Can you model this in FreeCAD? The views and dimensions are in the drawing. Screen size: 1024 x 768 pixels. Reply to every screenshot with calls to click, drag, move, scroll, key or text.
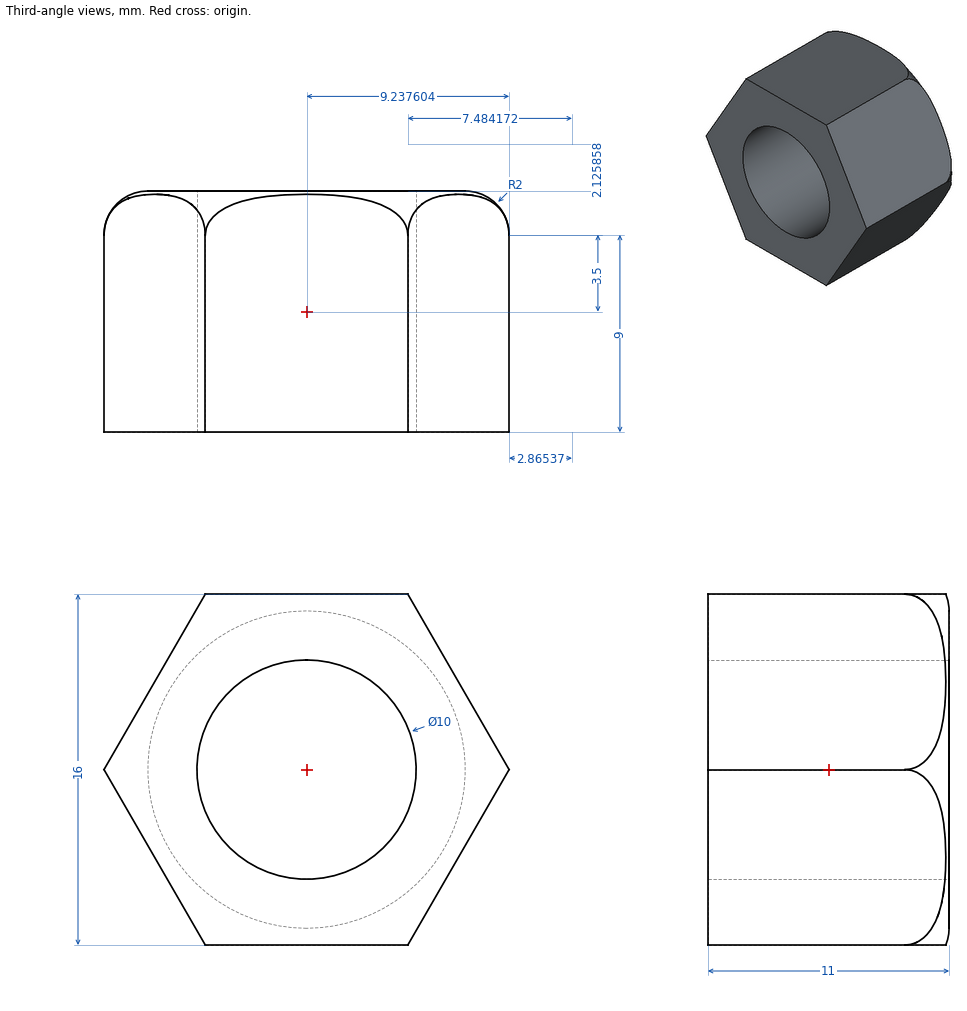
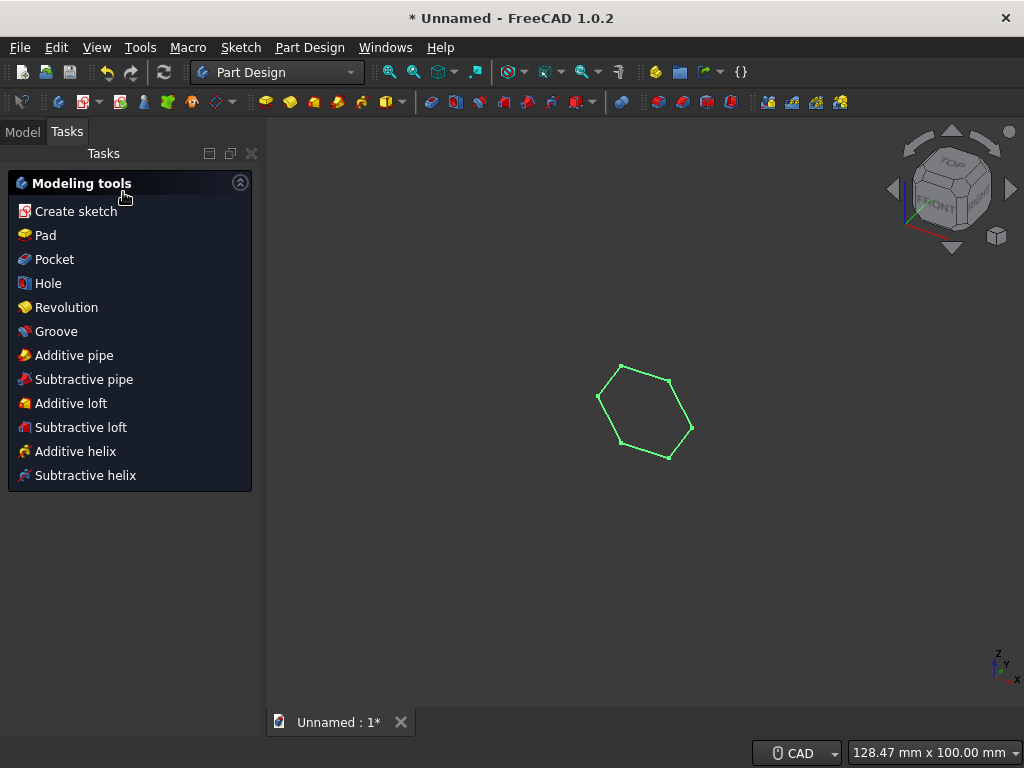
click(266, 102)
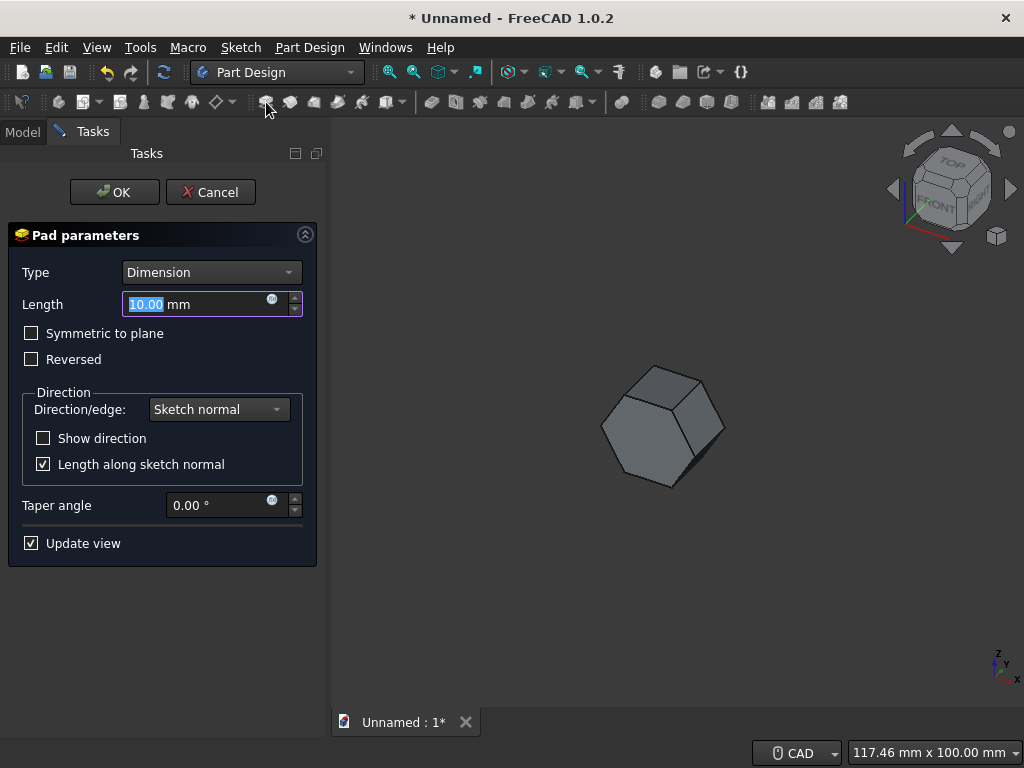
text(11)
key(Tab)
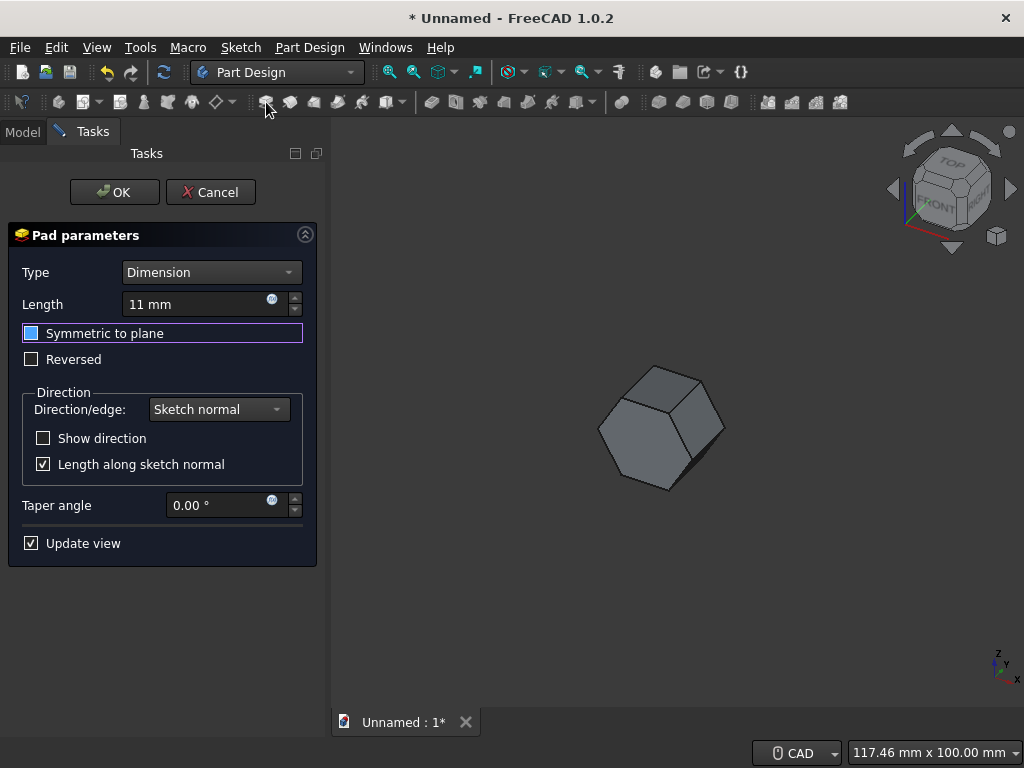
click(30, 333)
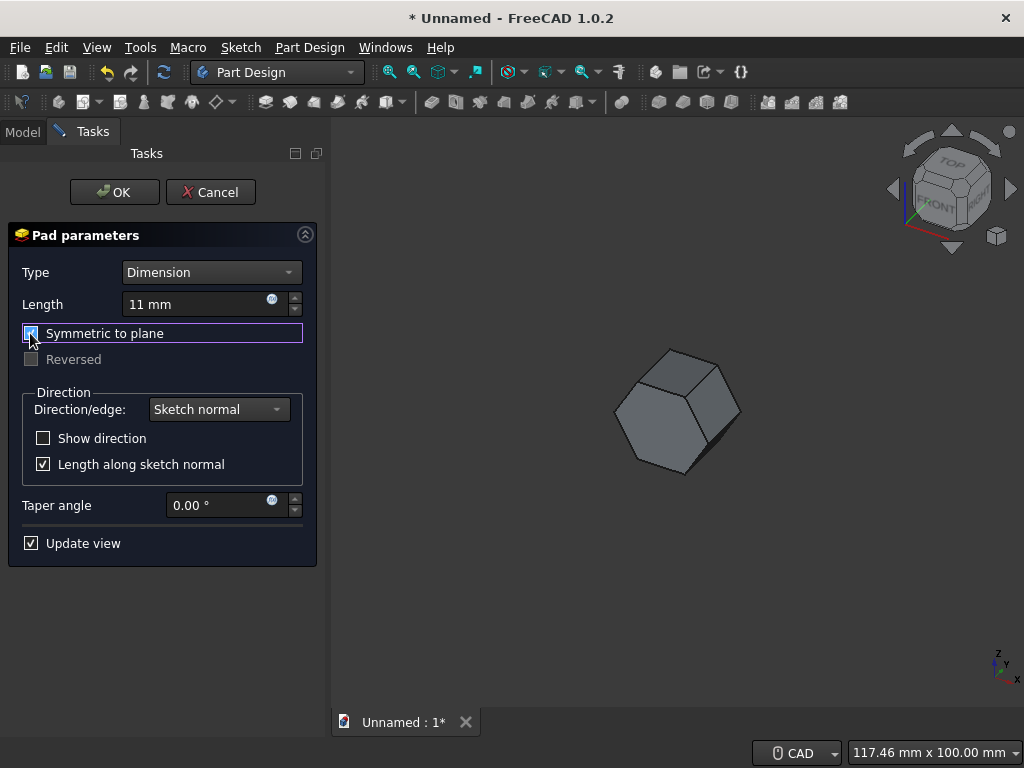
click(115, 192)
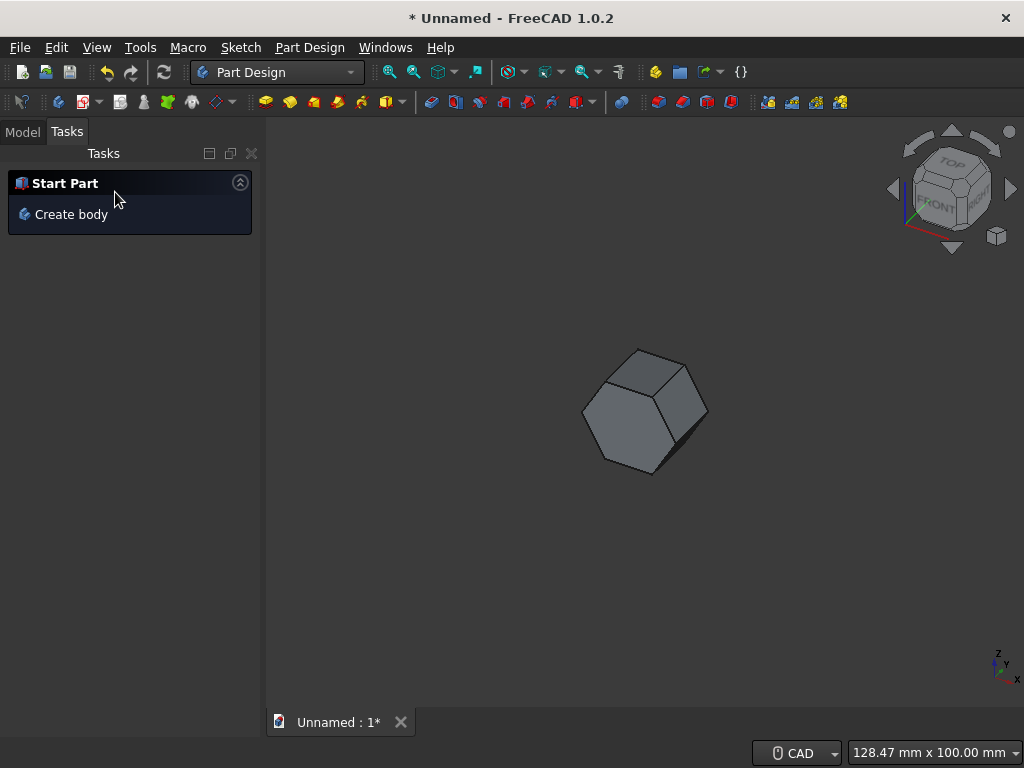
click(390, 72)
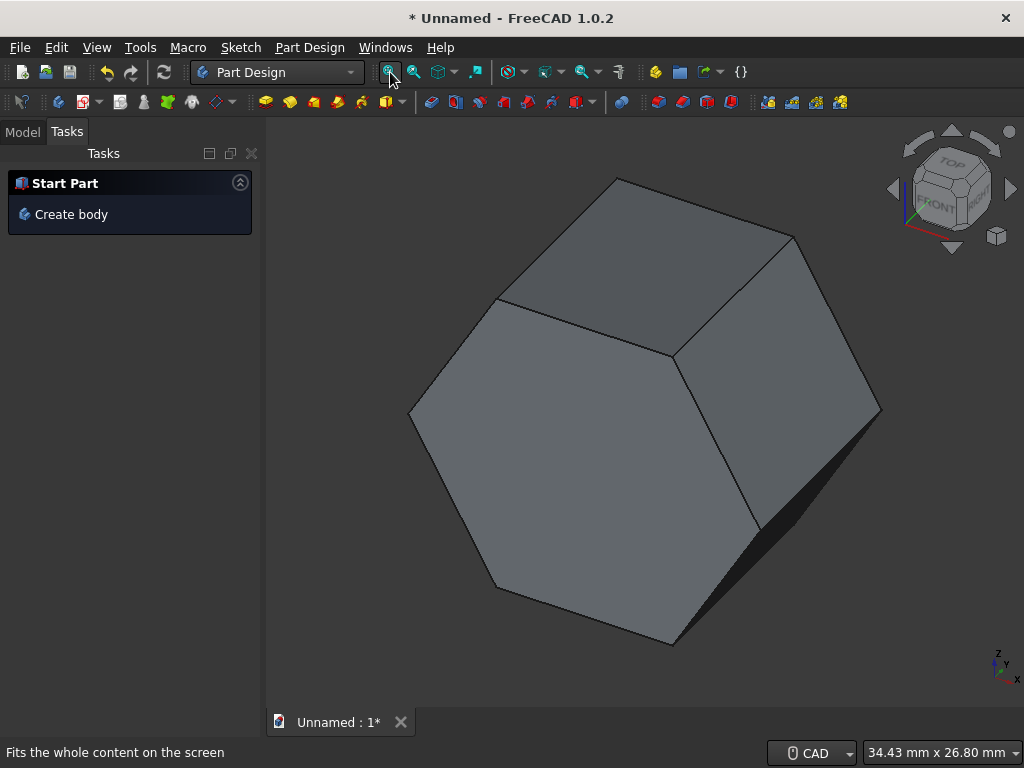
click(84, 102)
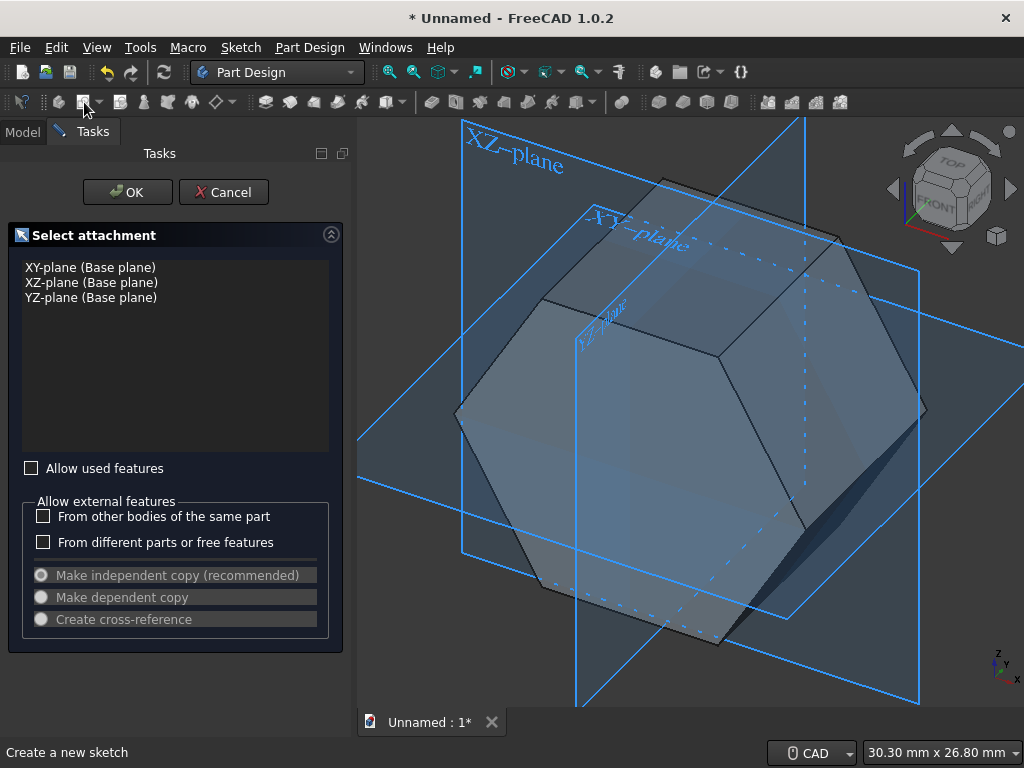
click(82, 268)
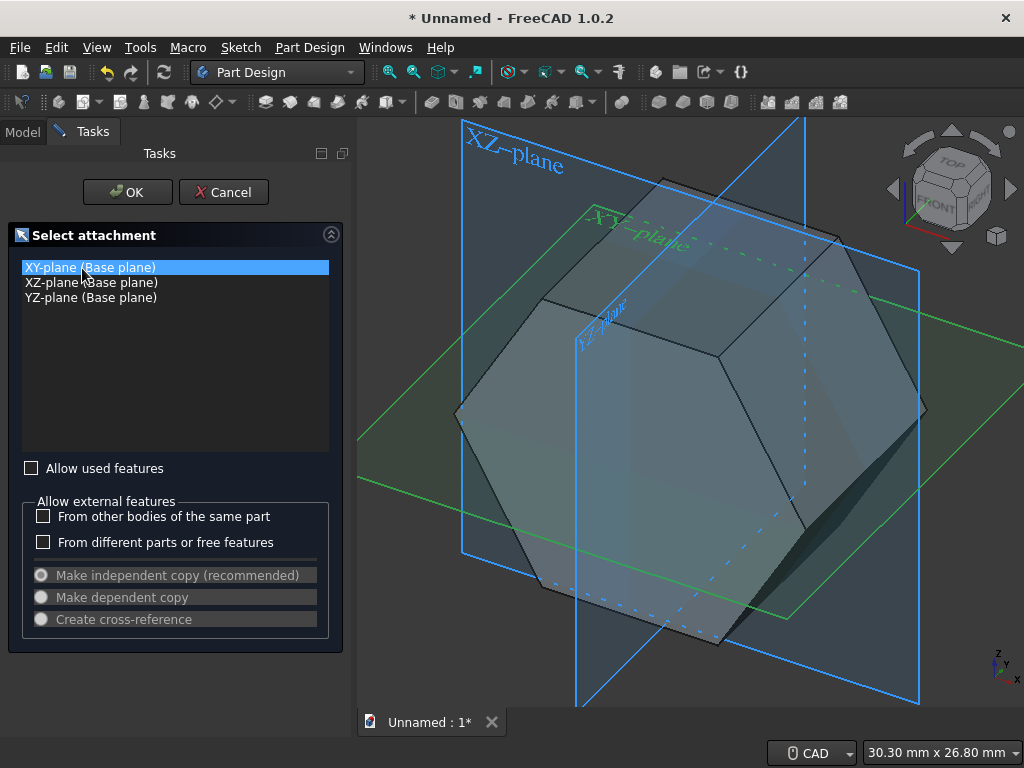
click(128, 192)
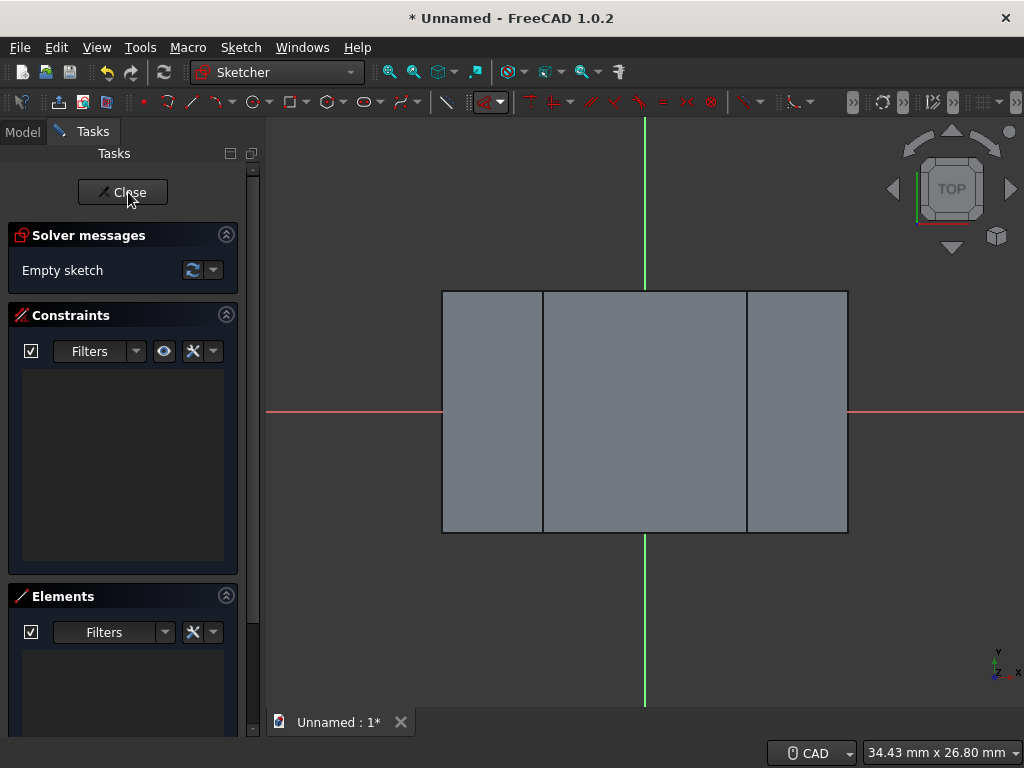
click(108, 102)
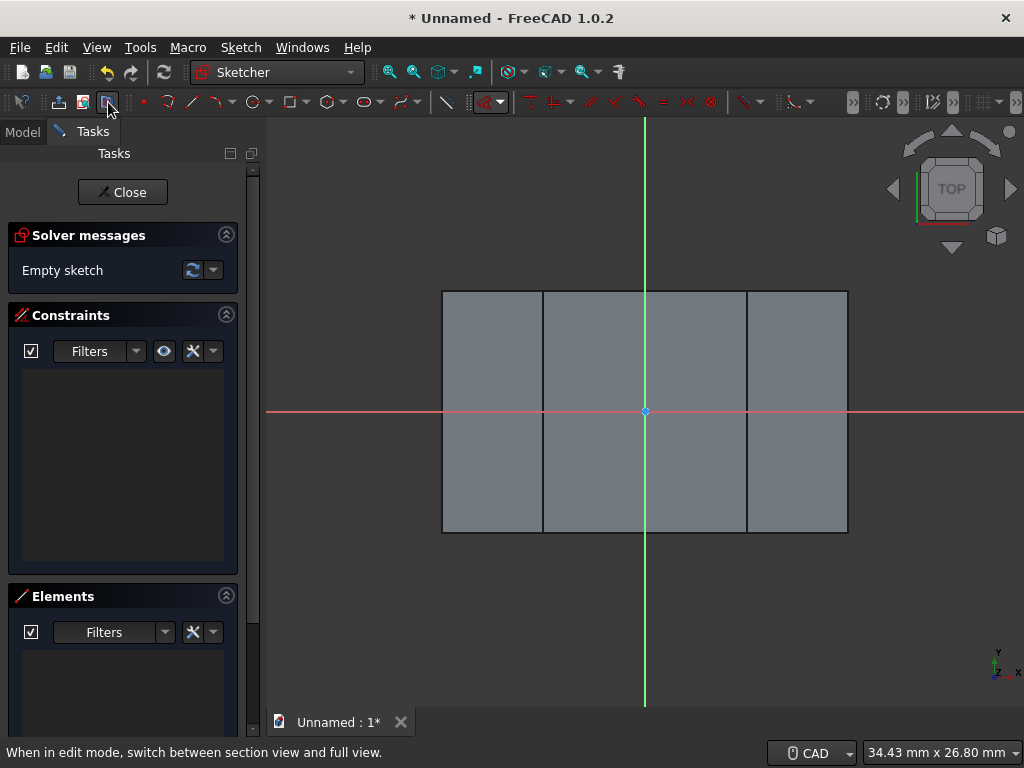
scroll(294, 518, down, 1)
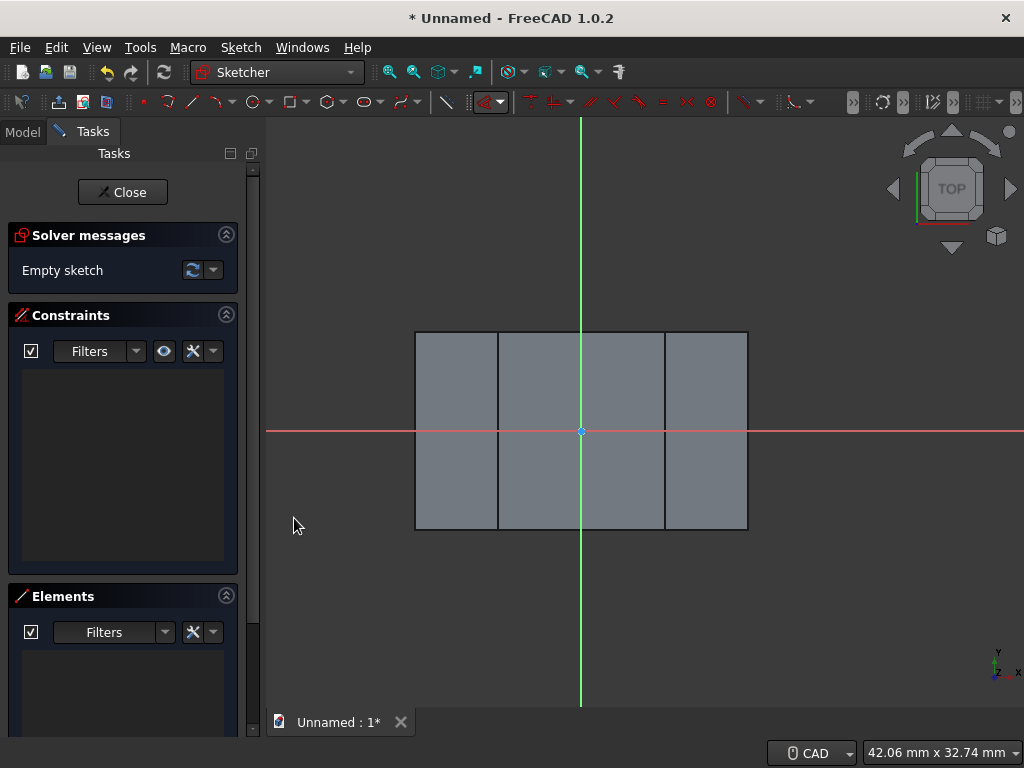
scroll(859, 413, up, 2)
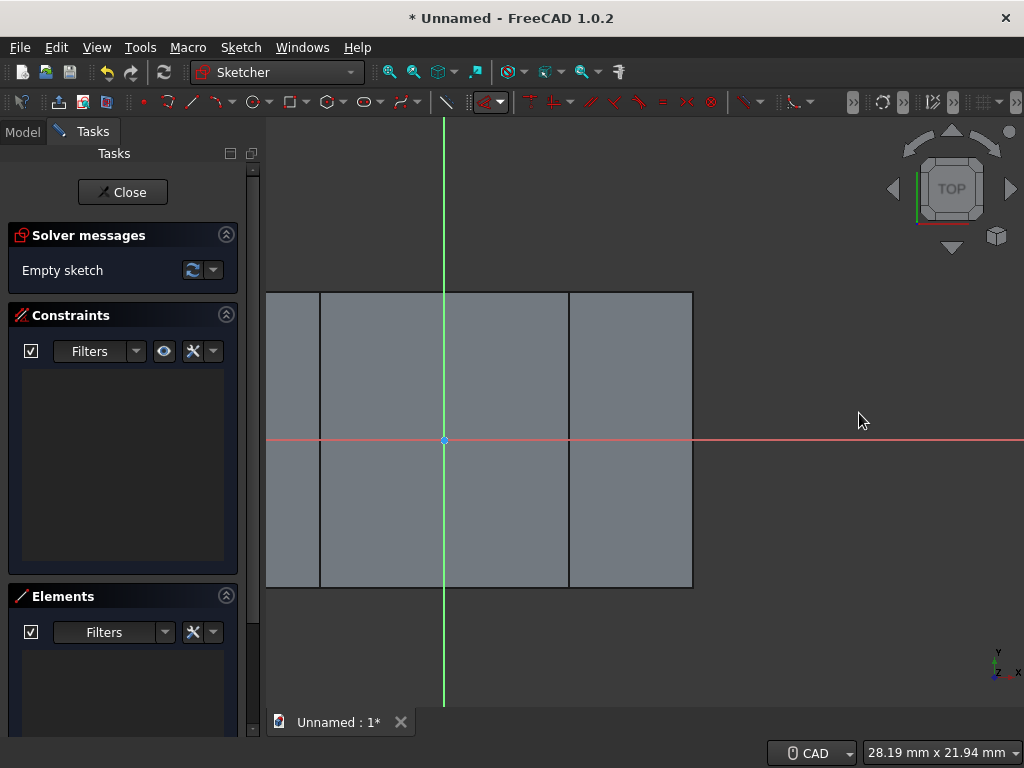
key(g)
key(m)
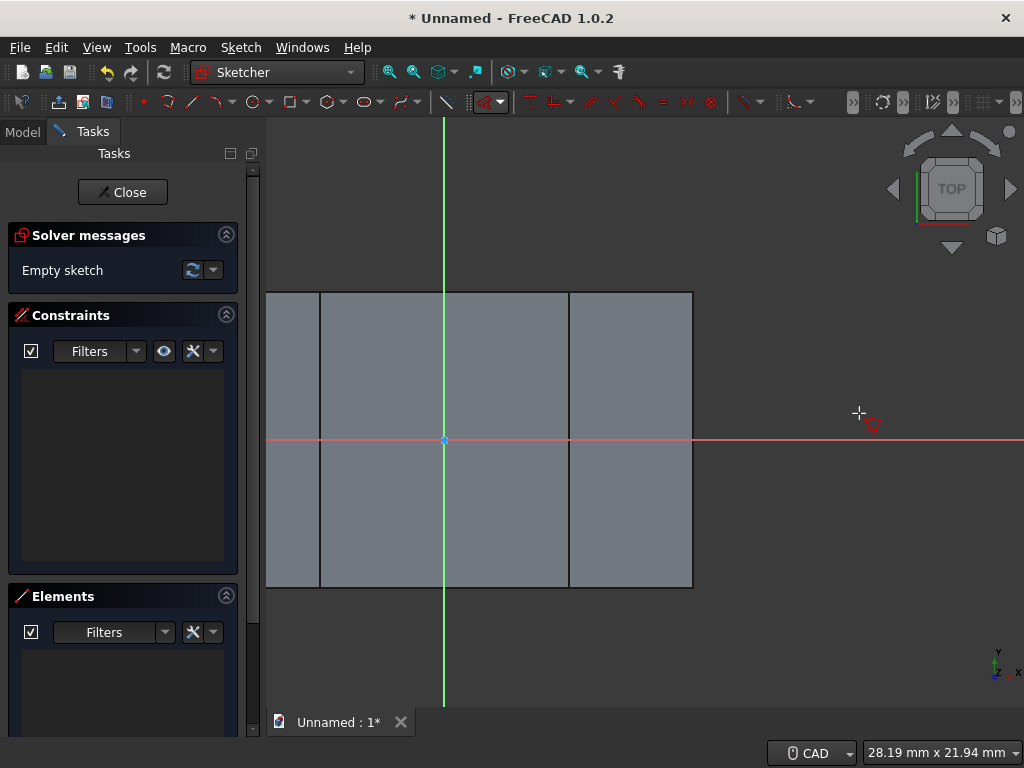
click(693, 346)
click(693, 588)
click(770, 588)
click(770, 235)
click(569, 235)
click(569, 292)
click(639, 292)
right_click(639, 292)